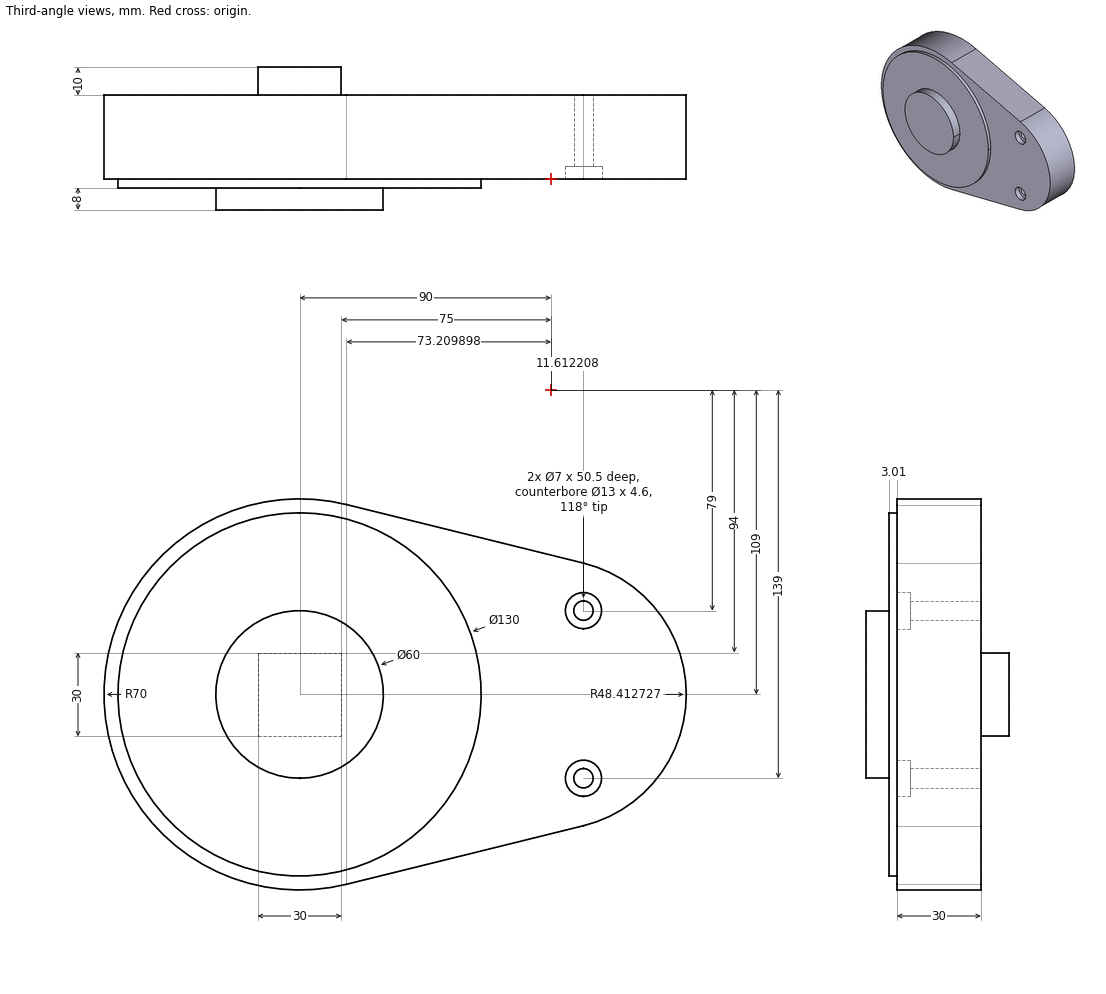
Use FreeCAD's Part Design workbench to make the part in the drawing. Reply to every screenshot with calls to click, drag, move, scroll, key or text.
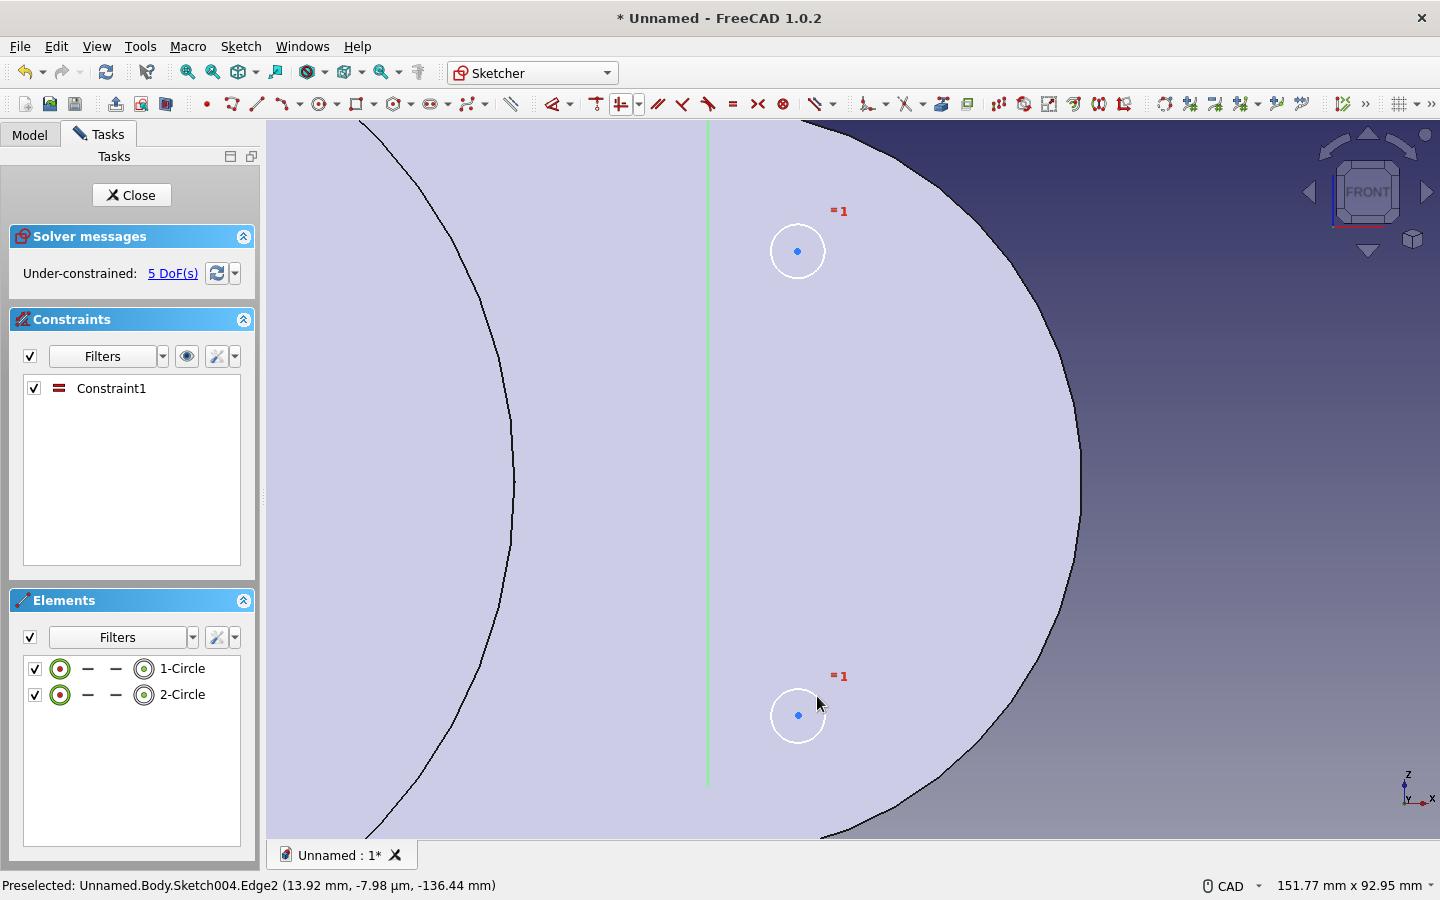
key(d)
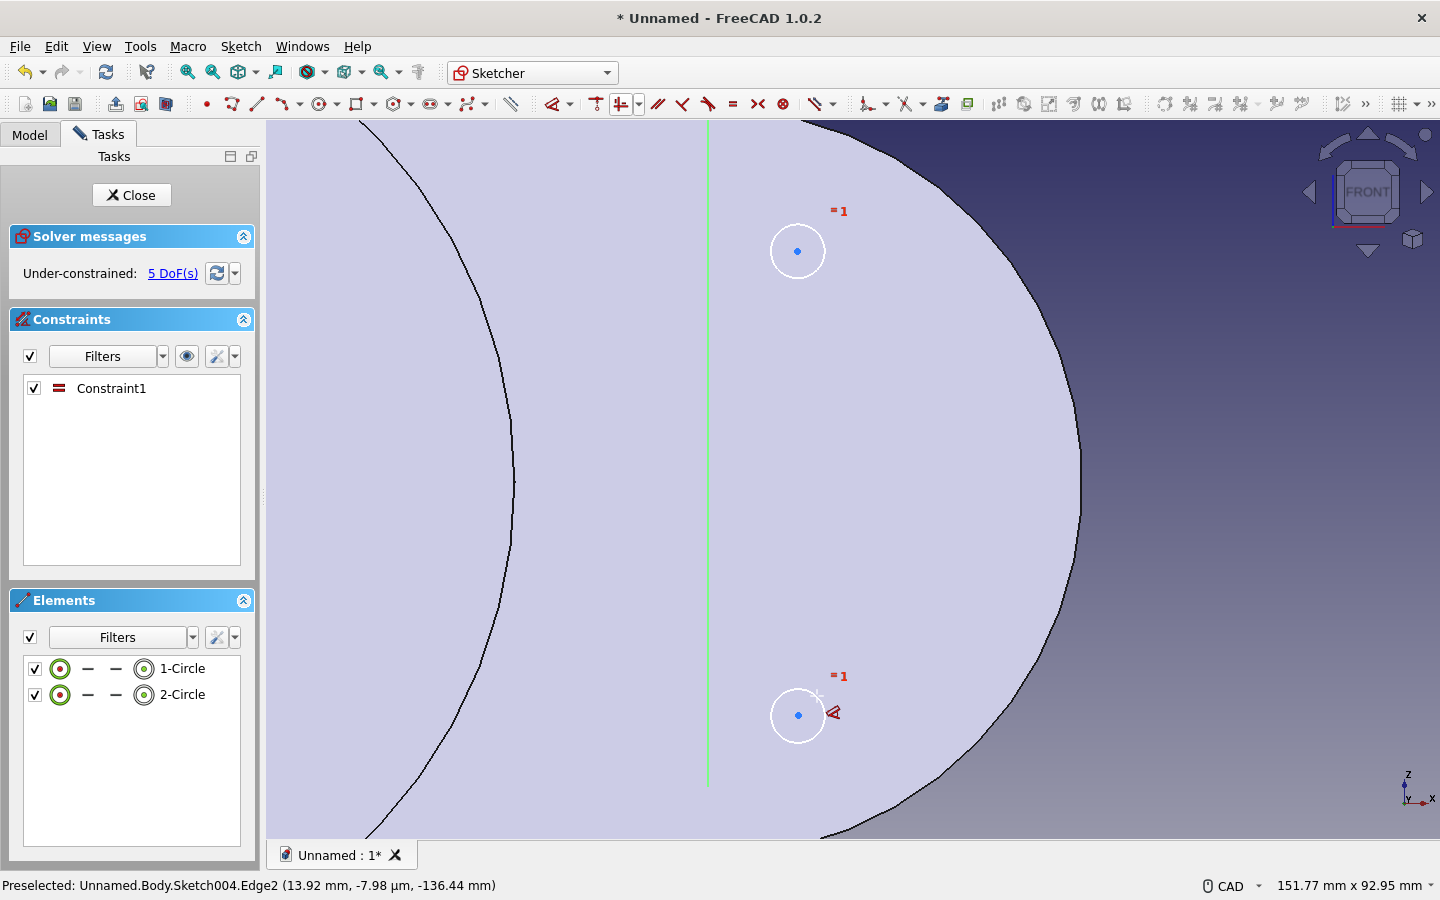
click(817, 232)
click(840, 209)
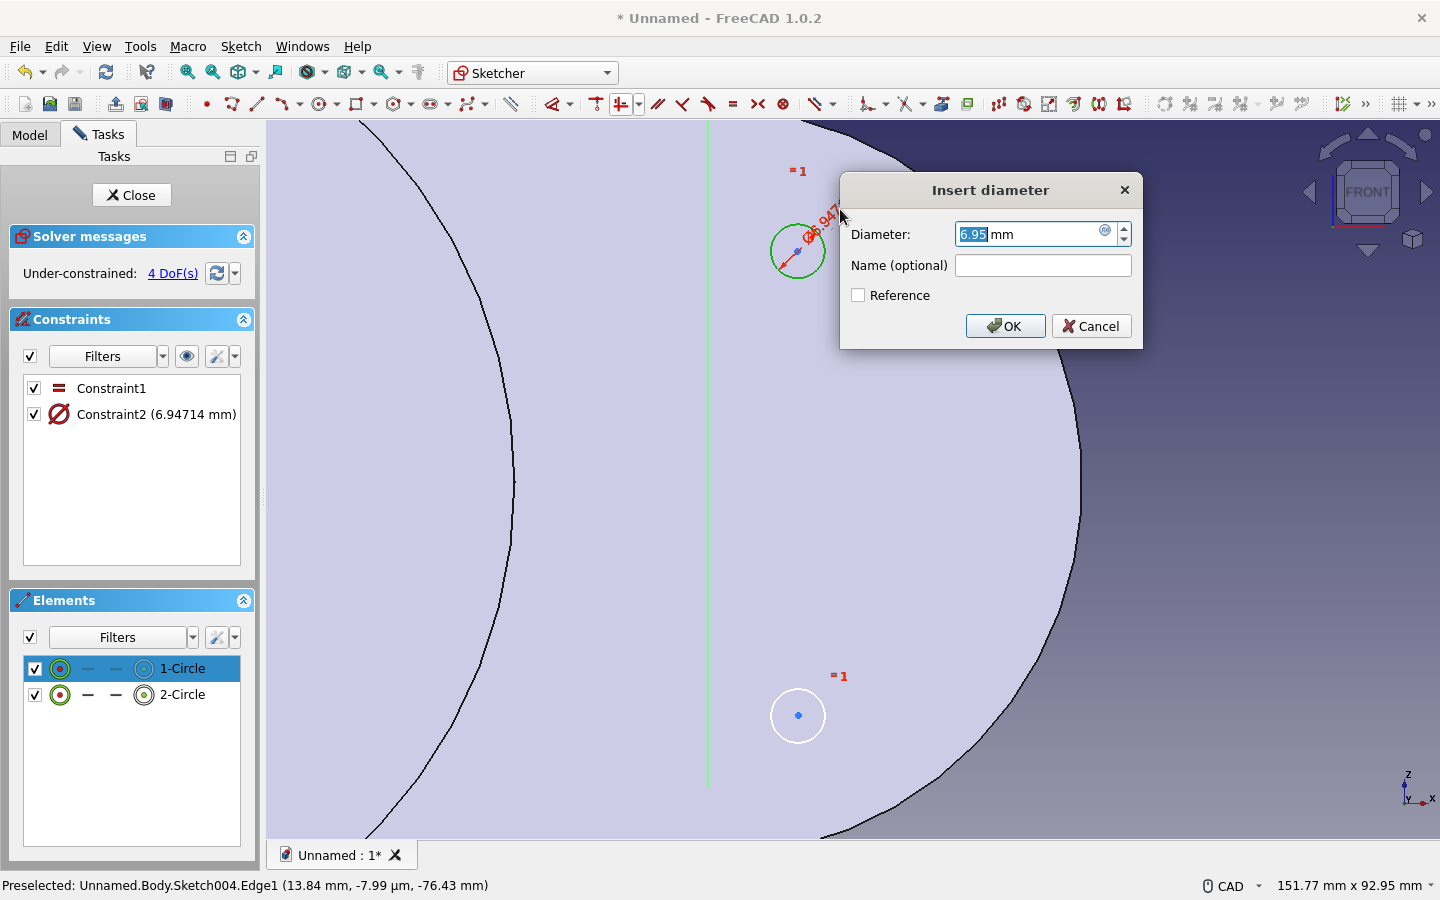
text(7)
key(Return)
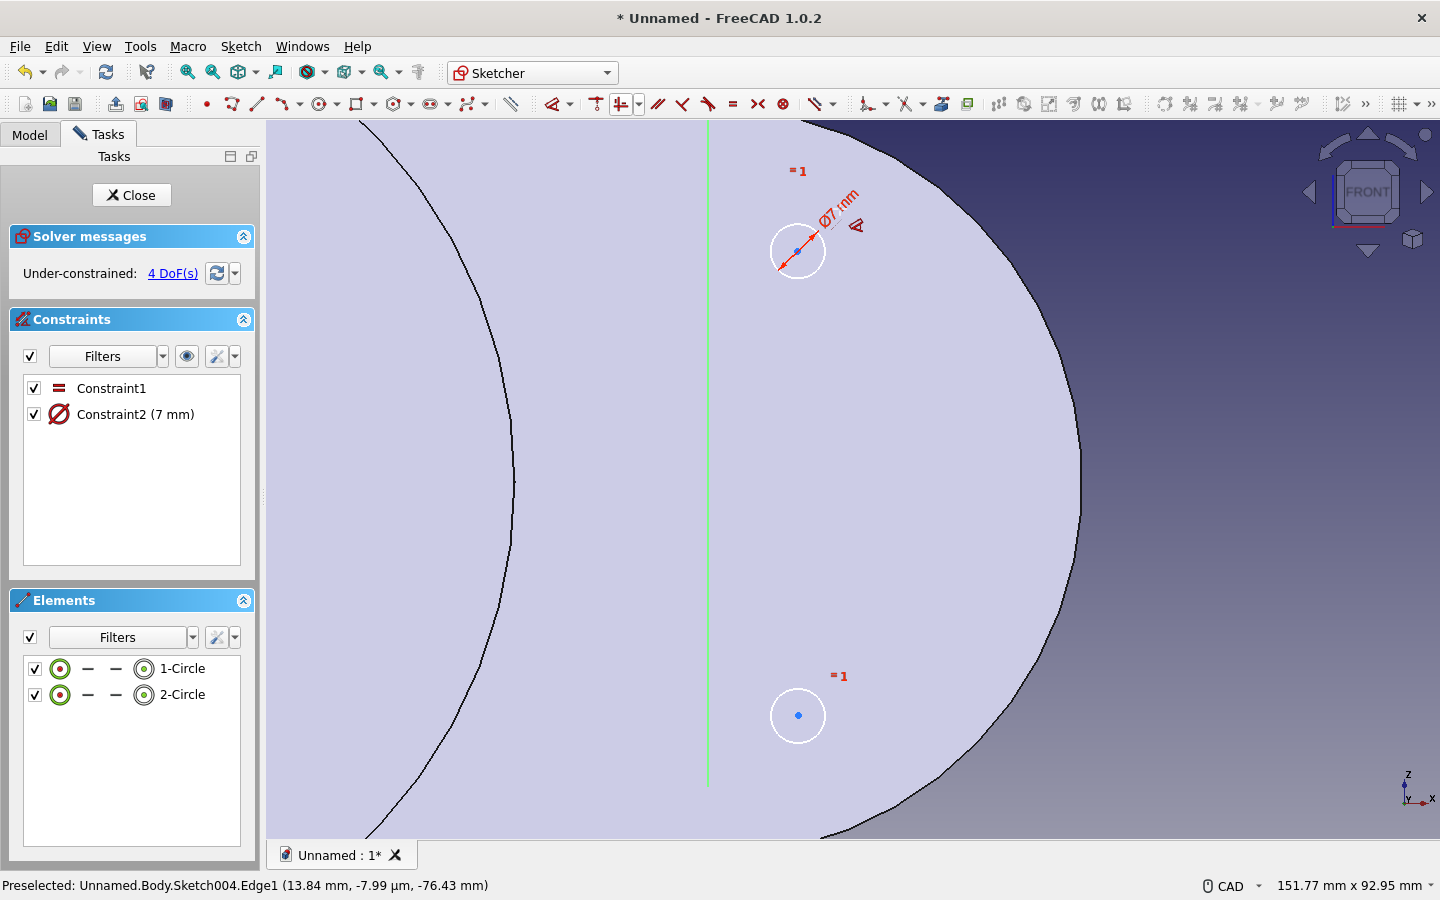
click(798, 251)
click(674, 200)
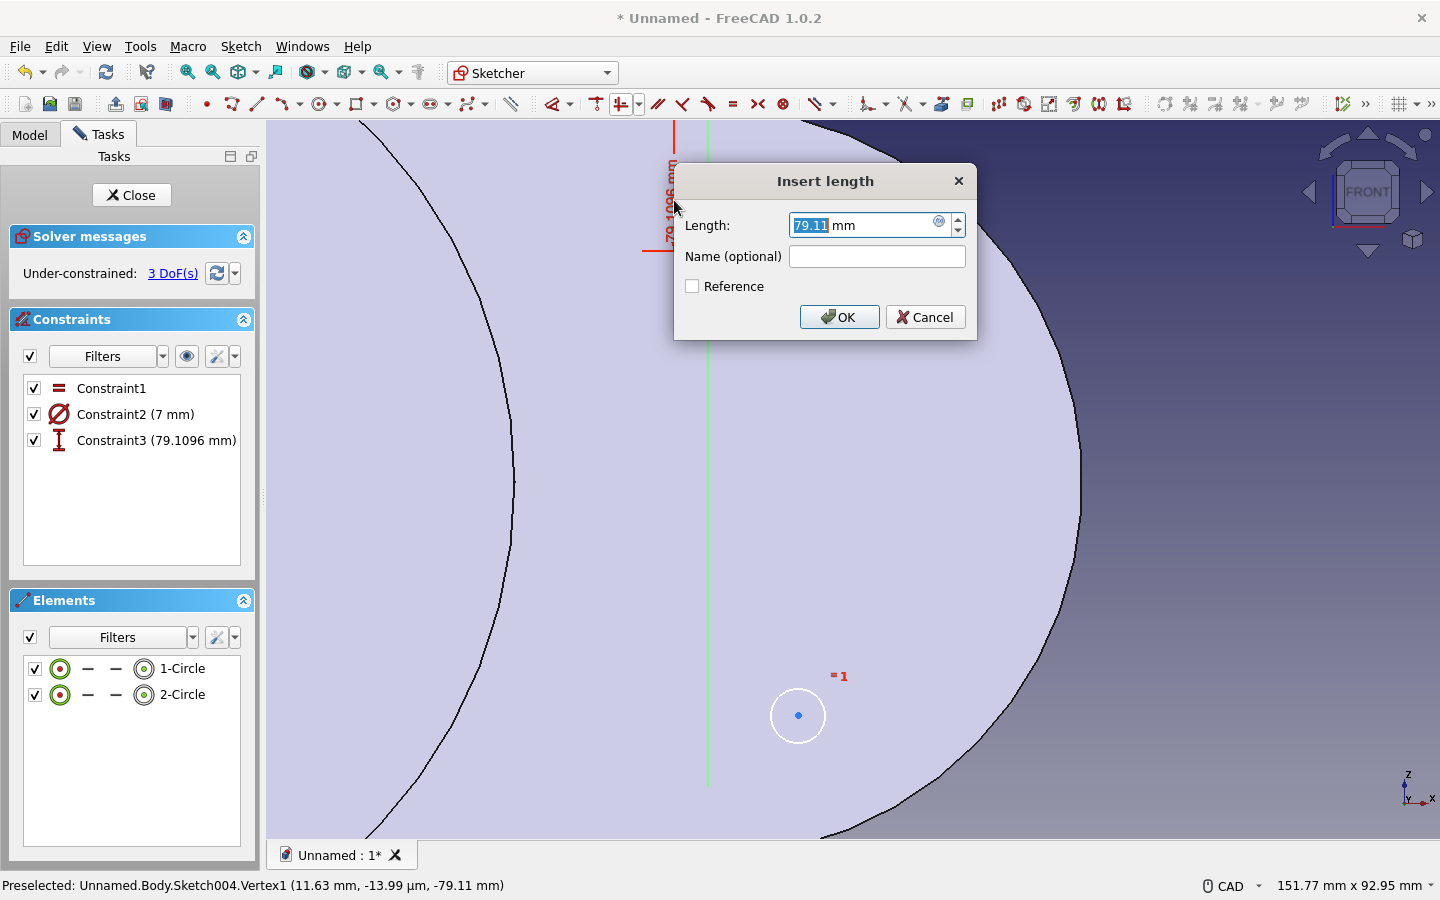
text(79)
key(Return)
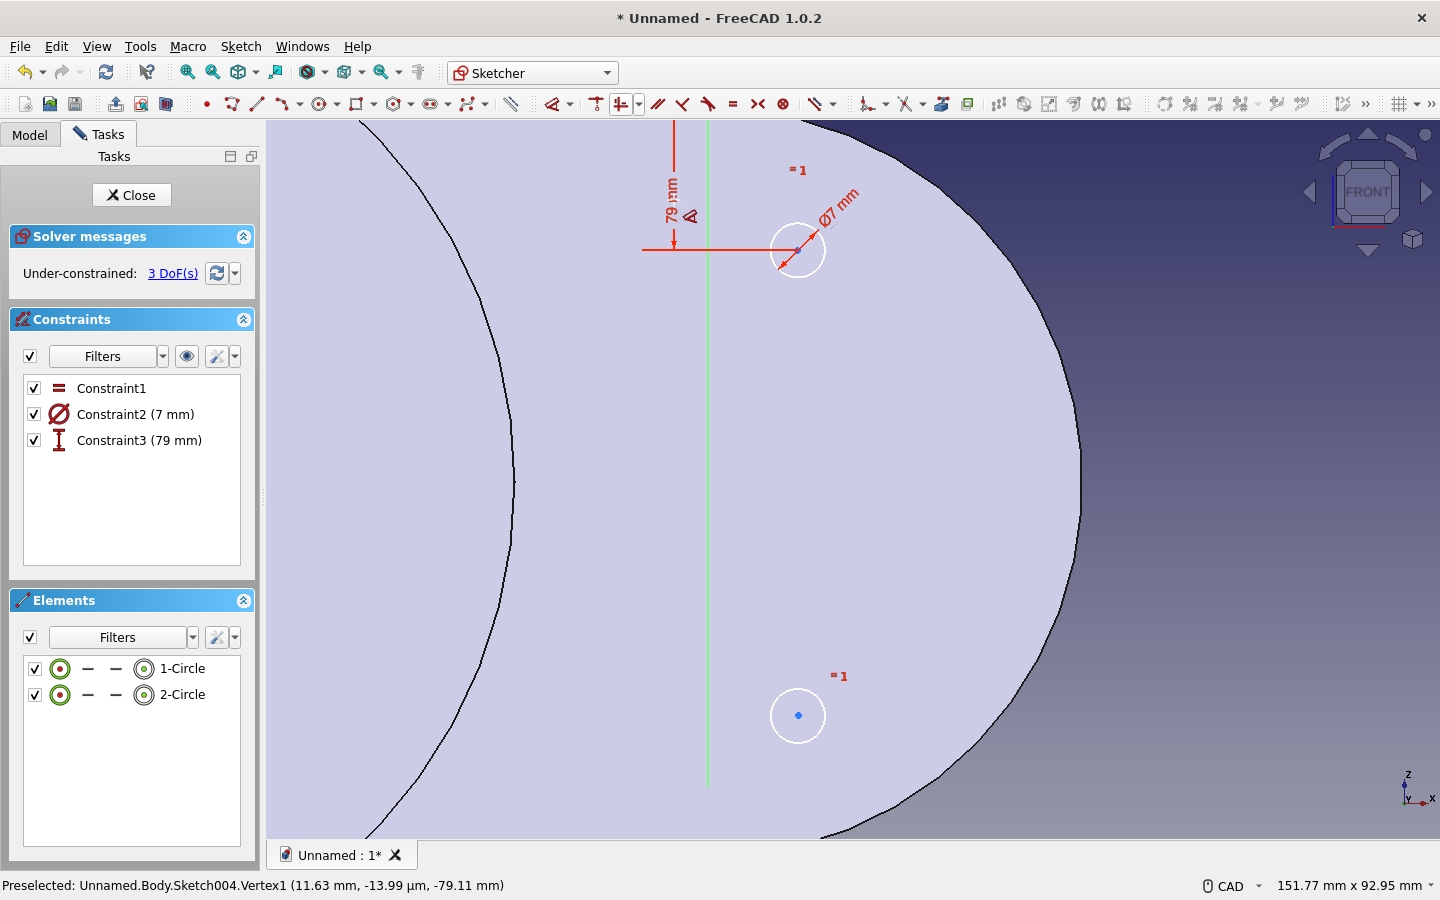
click(798, 716)
click(674, 432)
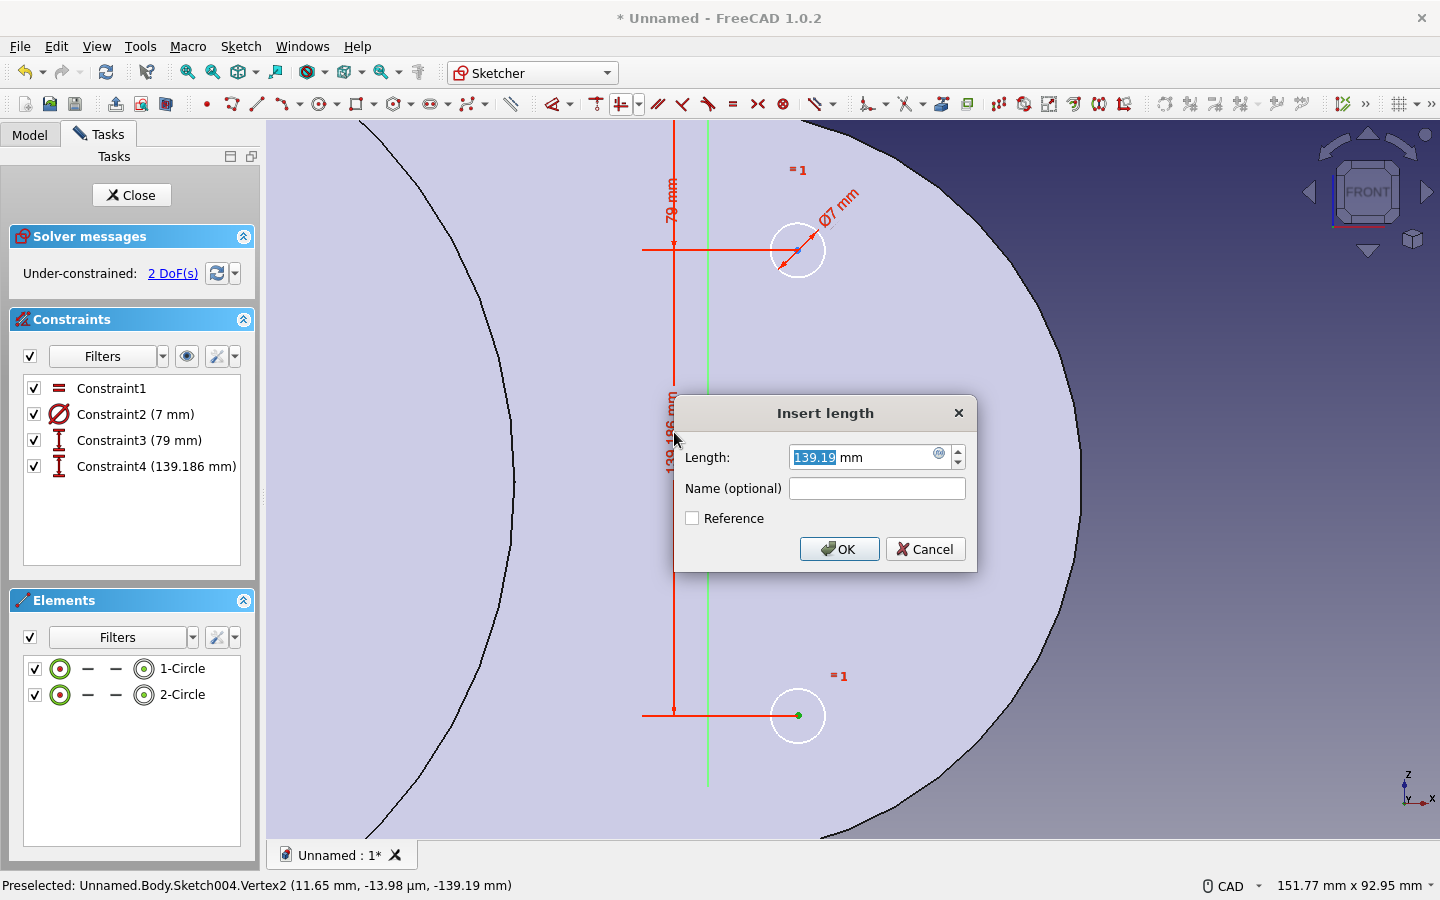
text(139)
key(Return)